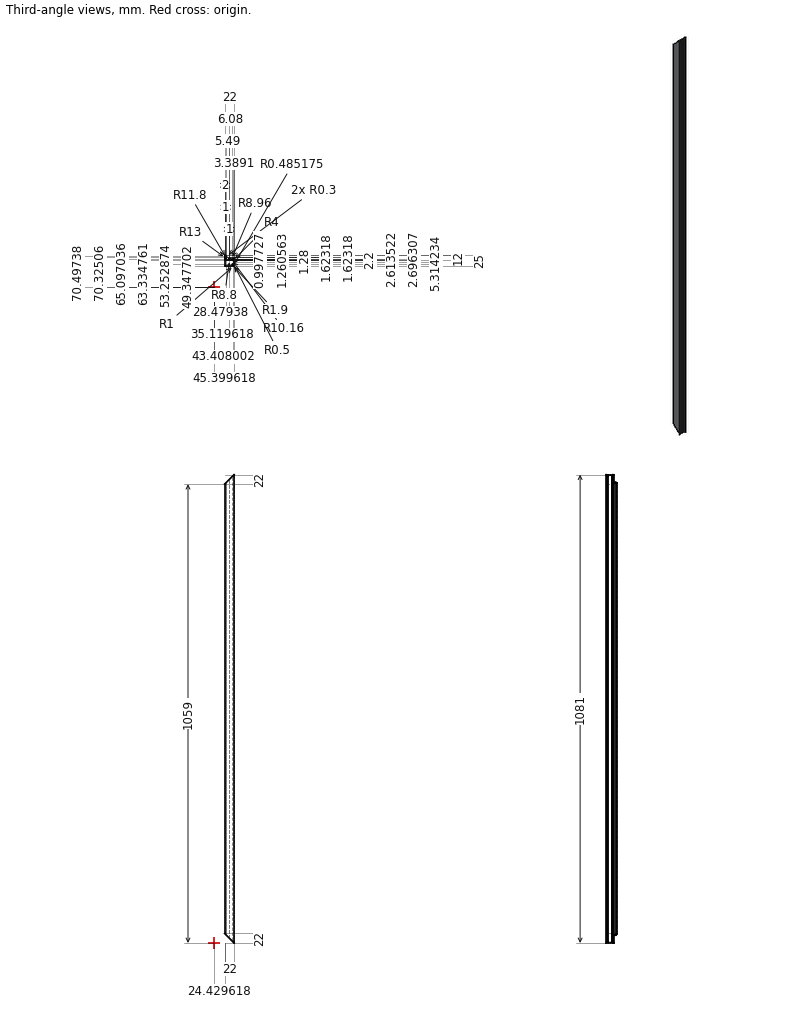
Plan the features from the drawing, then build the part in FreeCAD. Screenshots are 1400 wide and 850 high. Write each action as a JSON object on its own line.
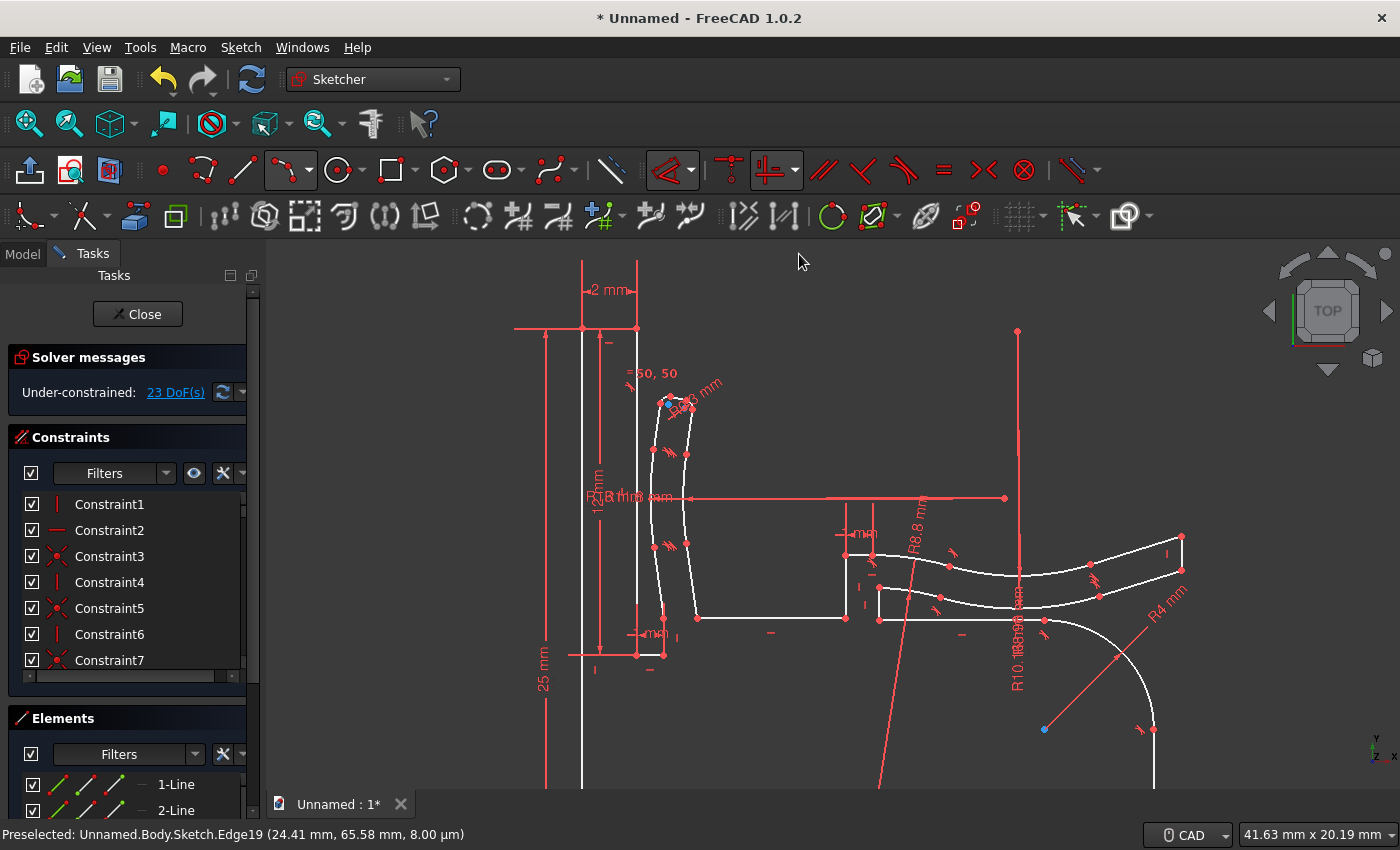
{"action": "scroll", "coordinate": [621, 328], "scroll_direction": "down", "scroll_amount": 3}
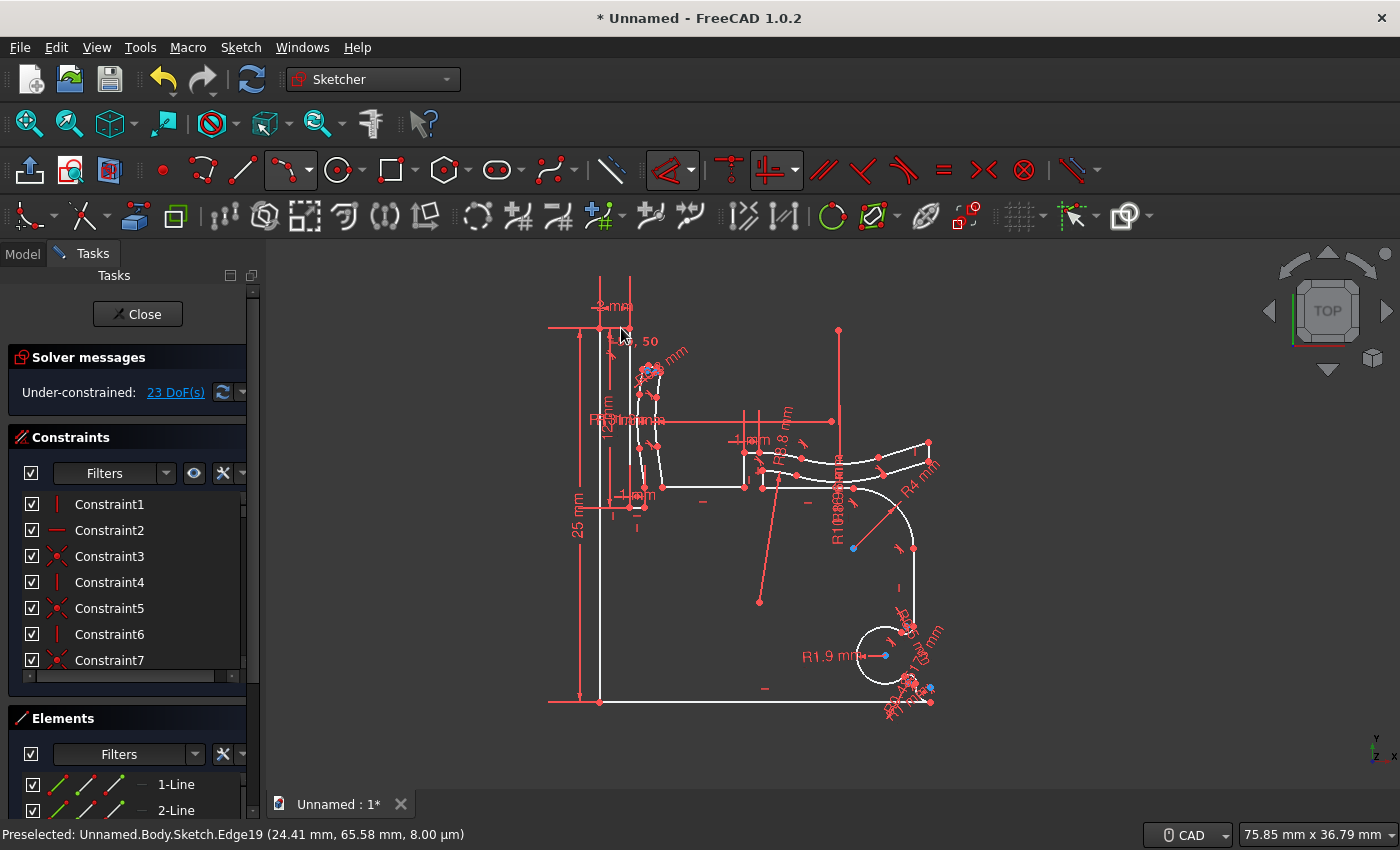
{"action": "left_click", "coordinate": [699, 702]}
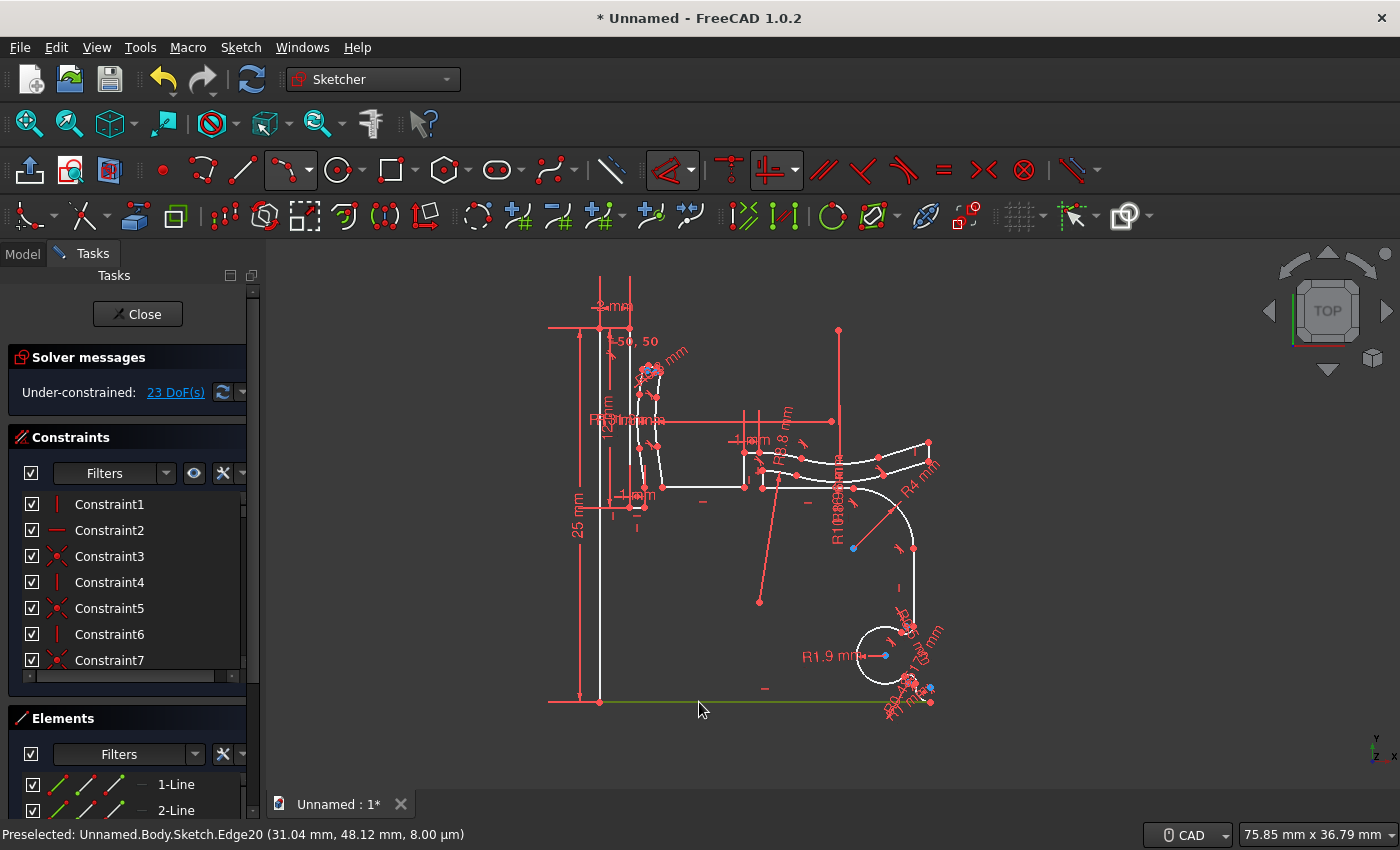
{"action": "key", "text": "l"}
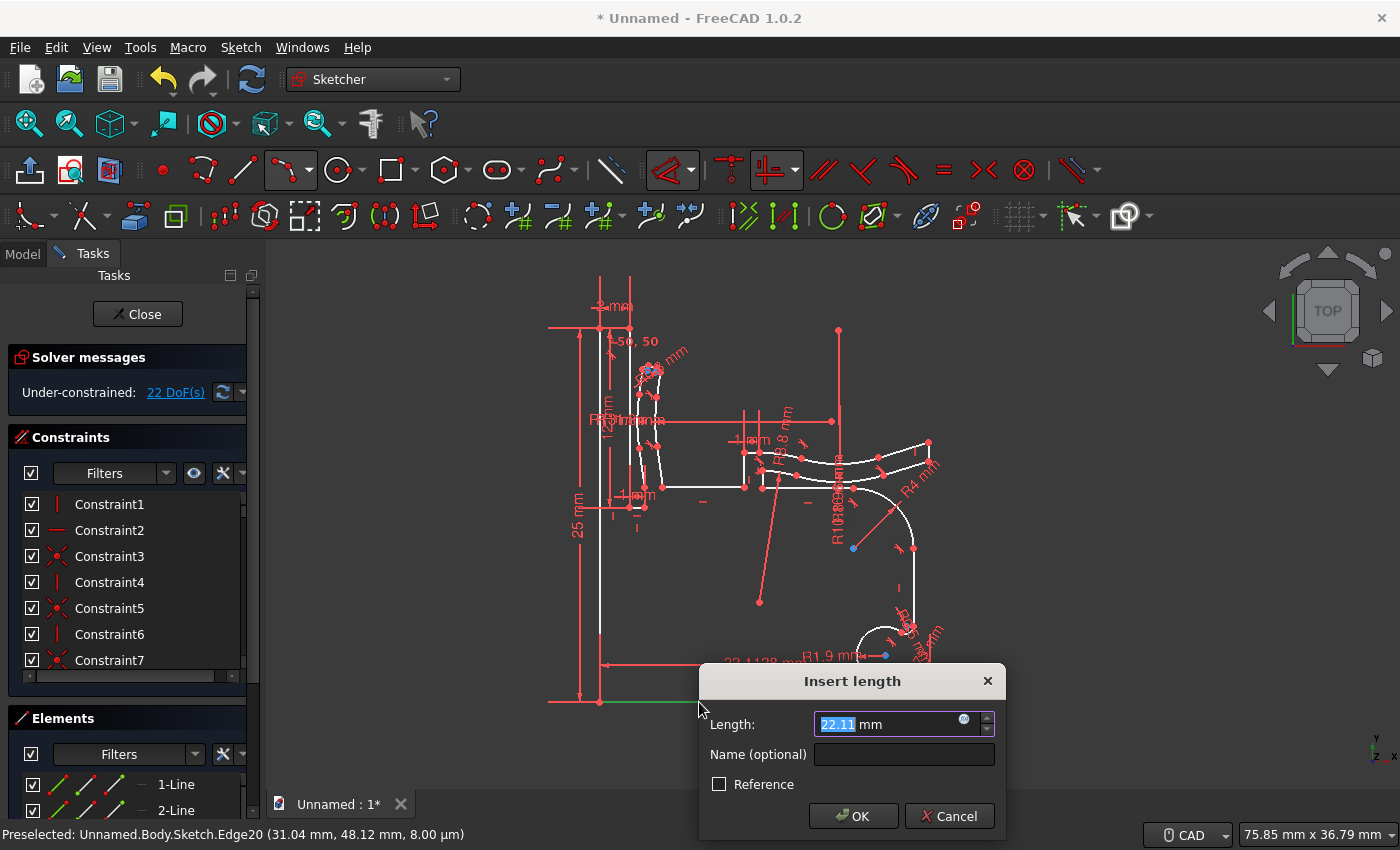
{"action": "type", "text": "22"}
{"action": "key", "text": "Return"}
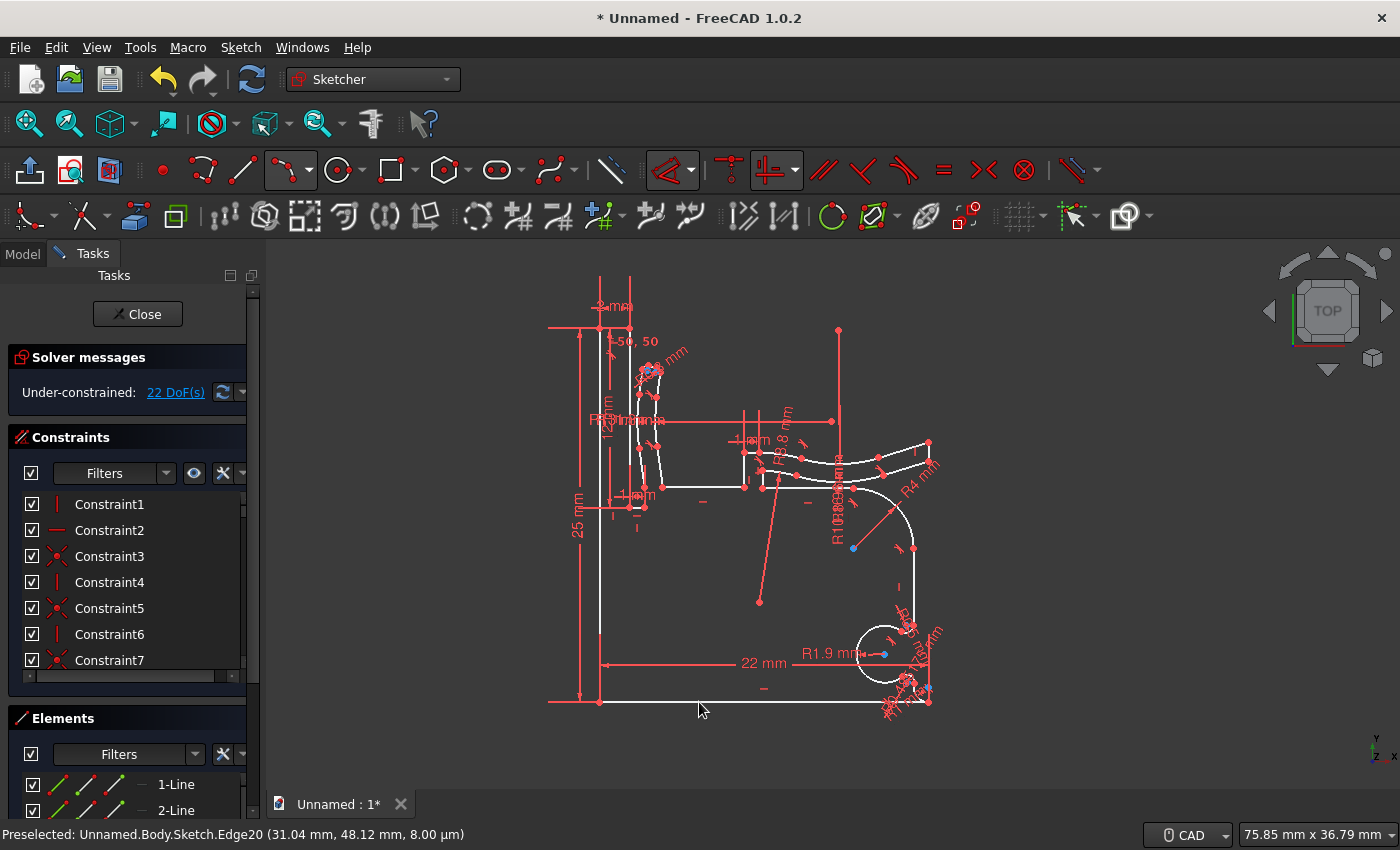
{"action": "scroll", "coordinate": [744, 463], "scroll_direction": "up", "scroll_amount": 2}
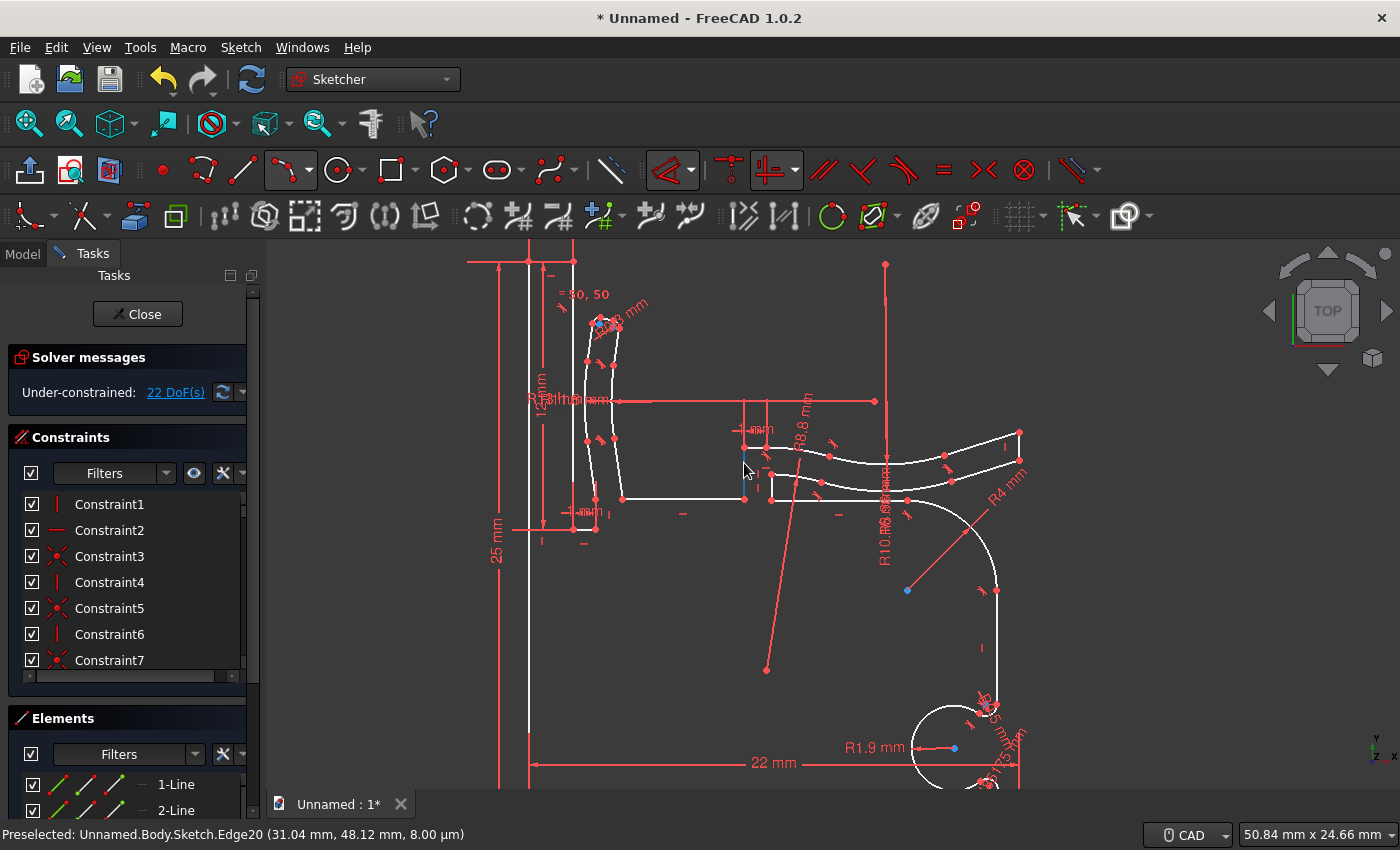
{"action": "left_click", "coordinate": [744, 463]}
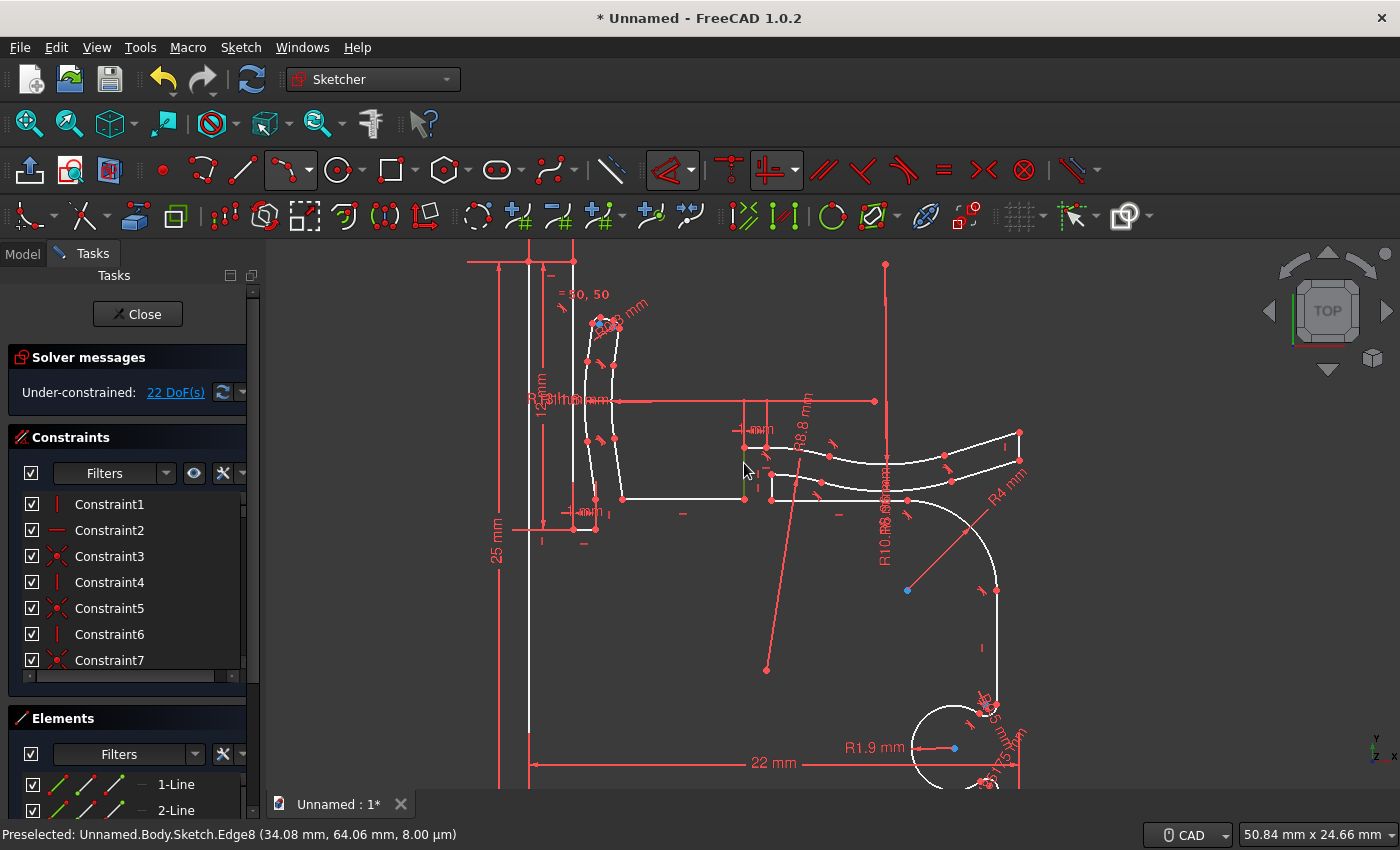
{"action": "key", "text": "i"}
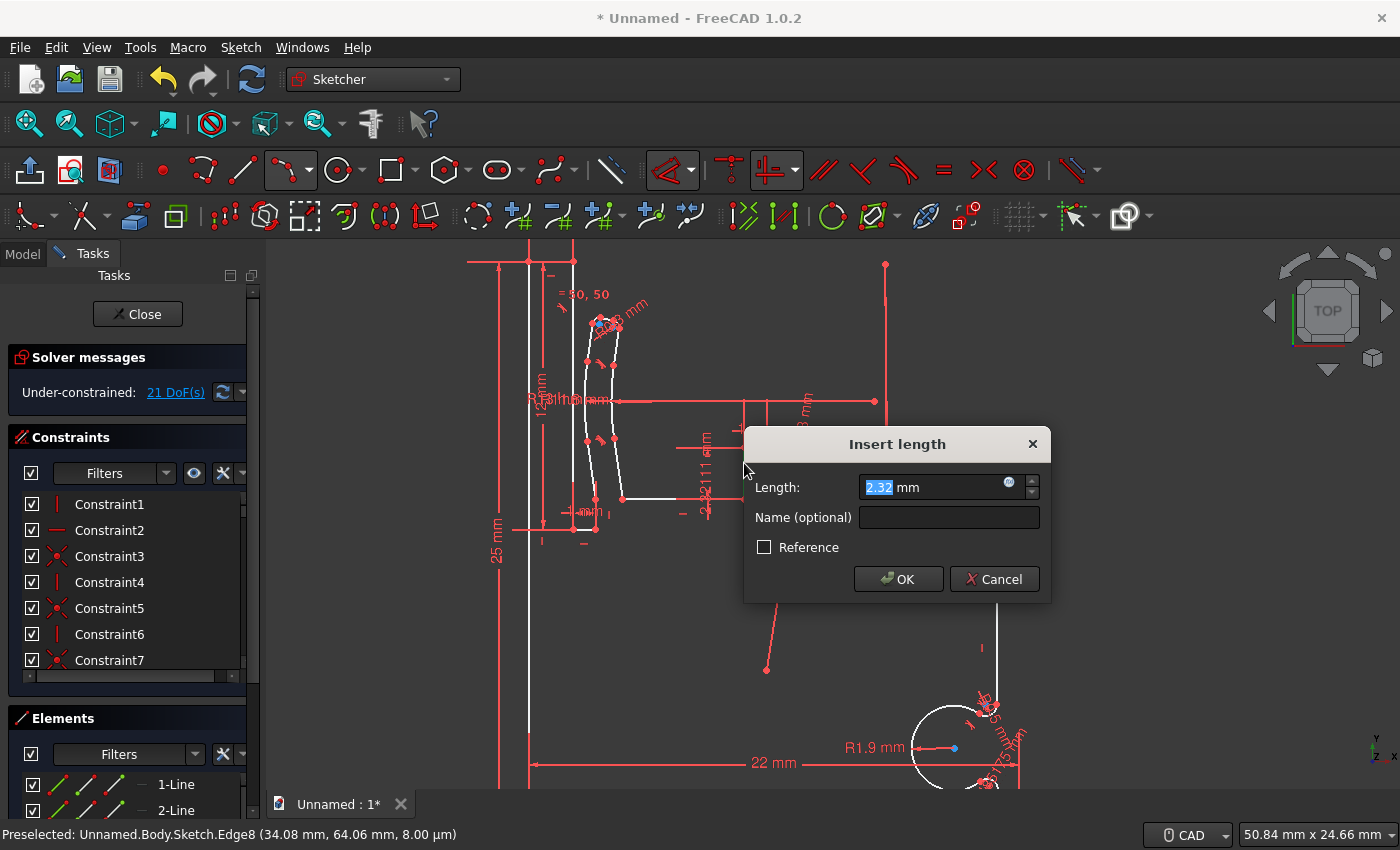
{"action": "type", "text": "2.2"}
{"action": "key", "text": "Return"}